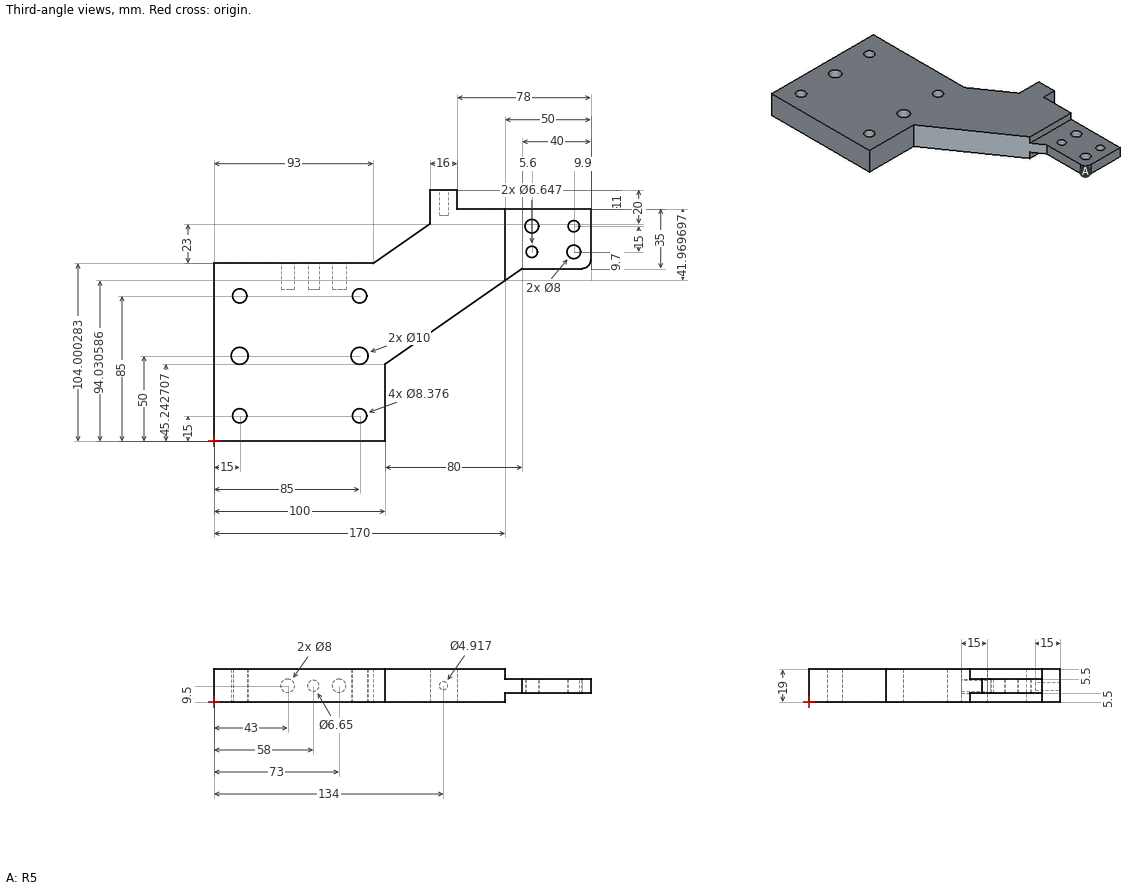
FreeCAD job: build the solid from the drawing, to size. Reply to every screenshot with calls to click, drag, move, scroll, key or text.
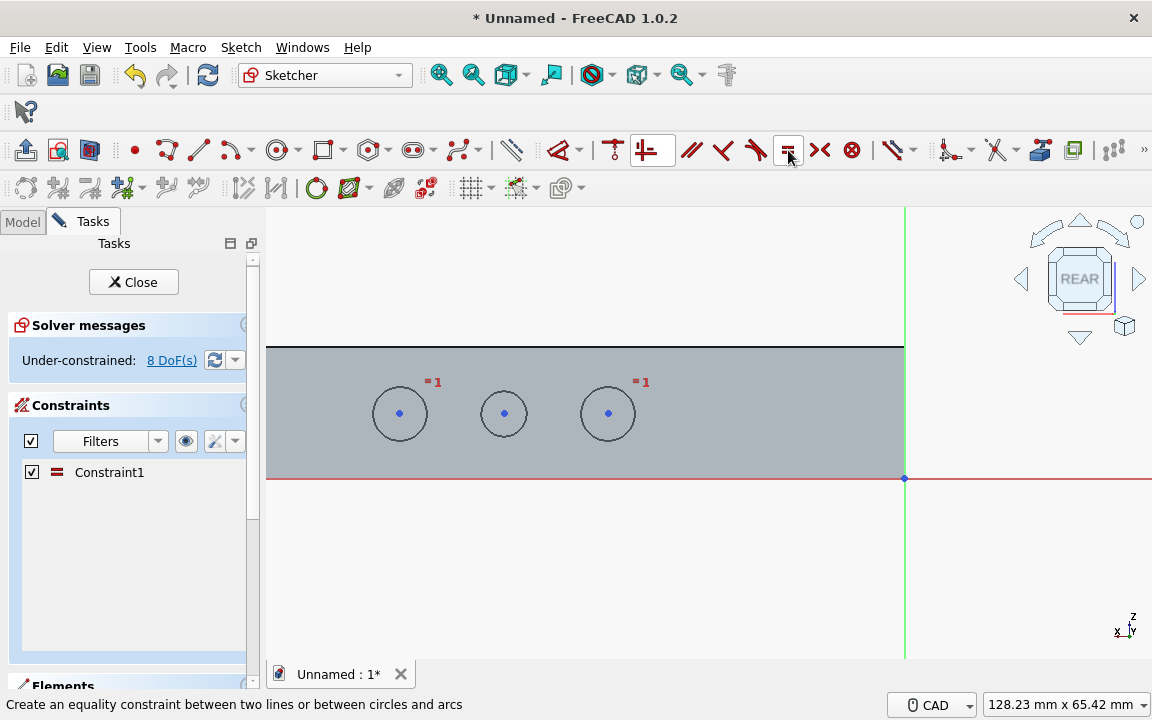
click(558, 150)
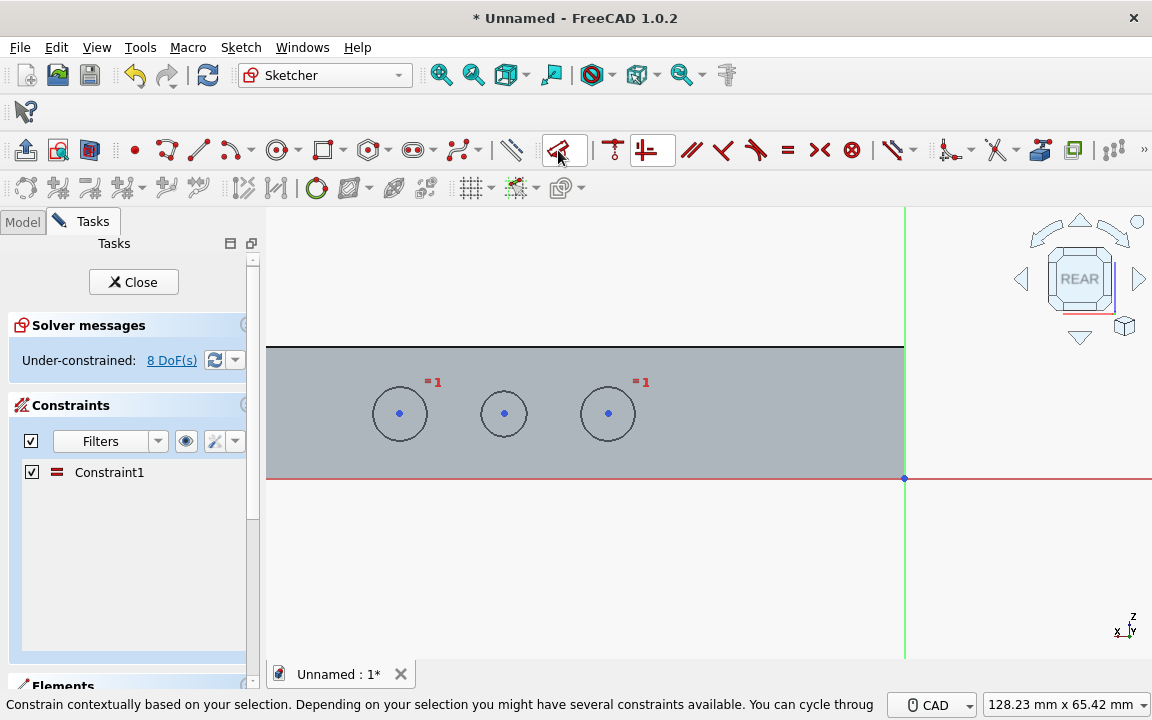
click(627, 395)
click(650, 372)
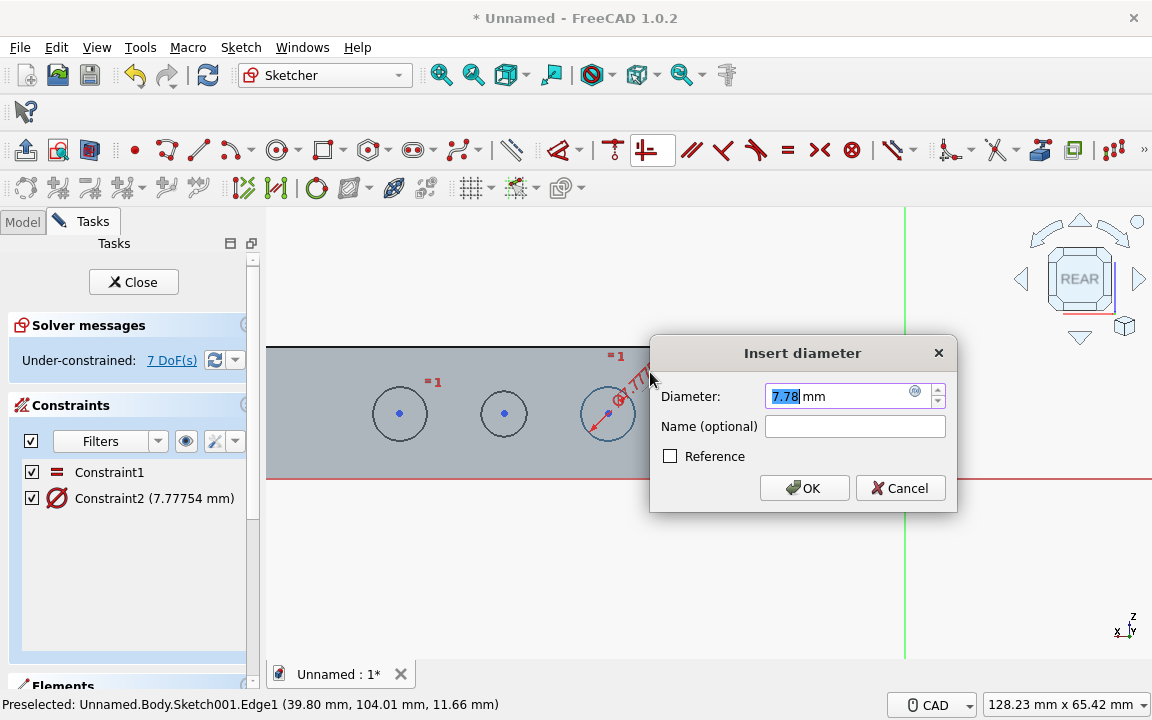
text(8)
key(Return)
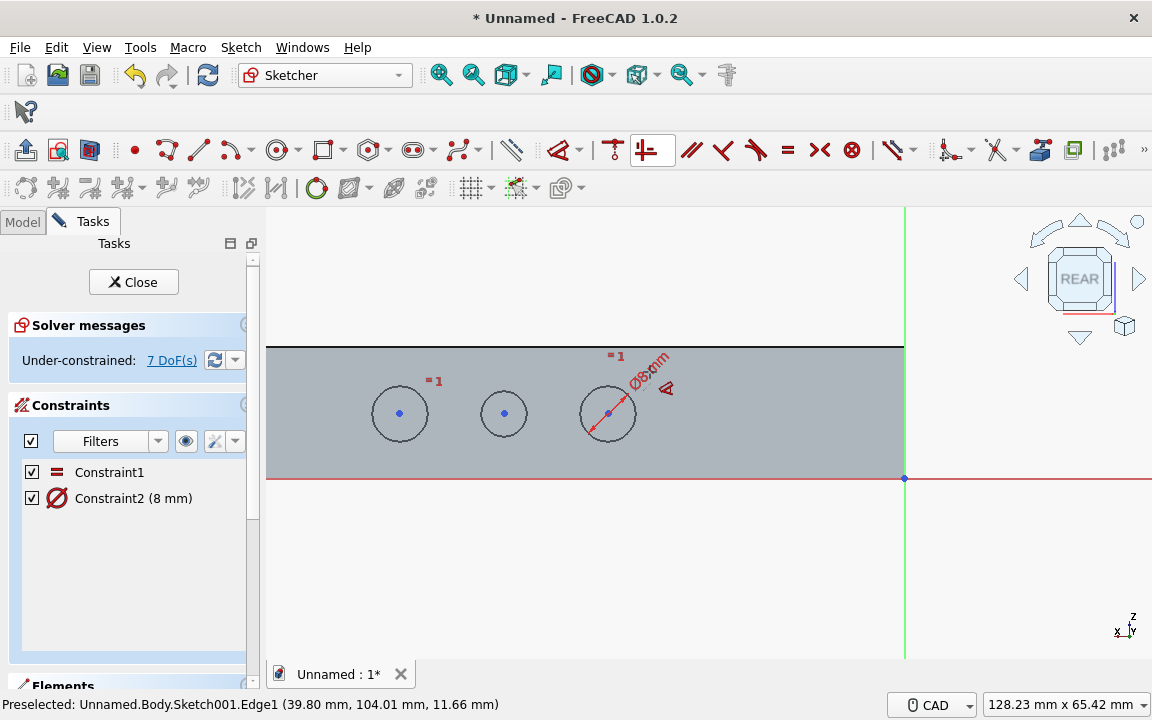
click(520, 398)
click(543, 375)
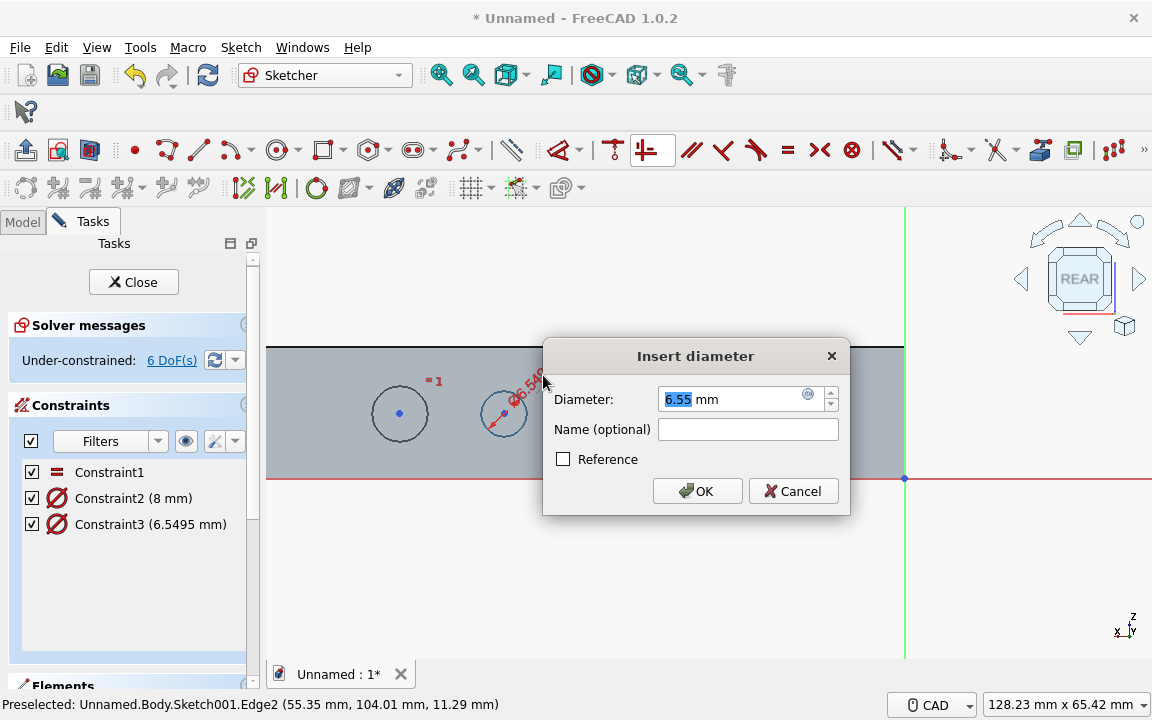
text(6.65)
key(Return)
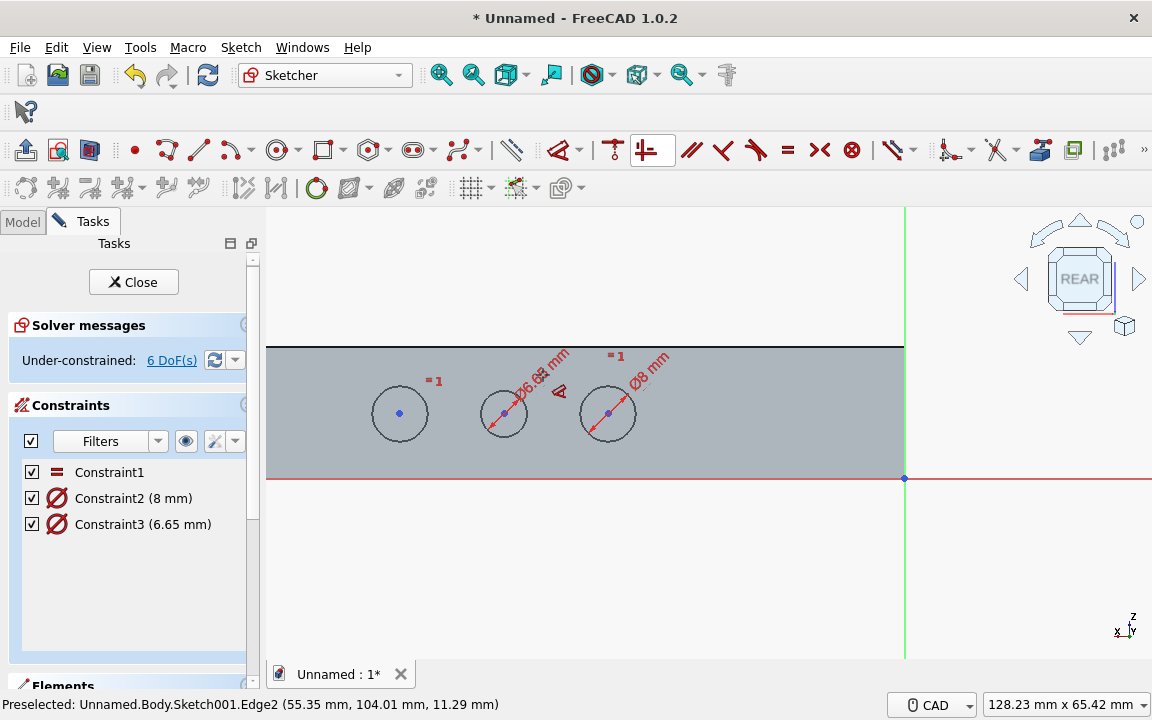
click(608, 414)
click(756, 513)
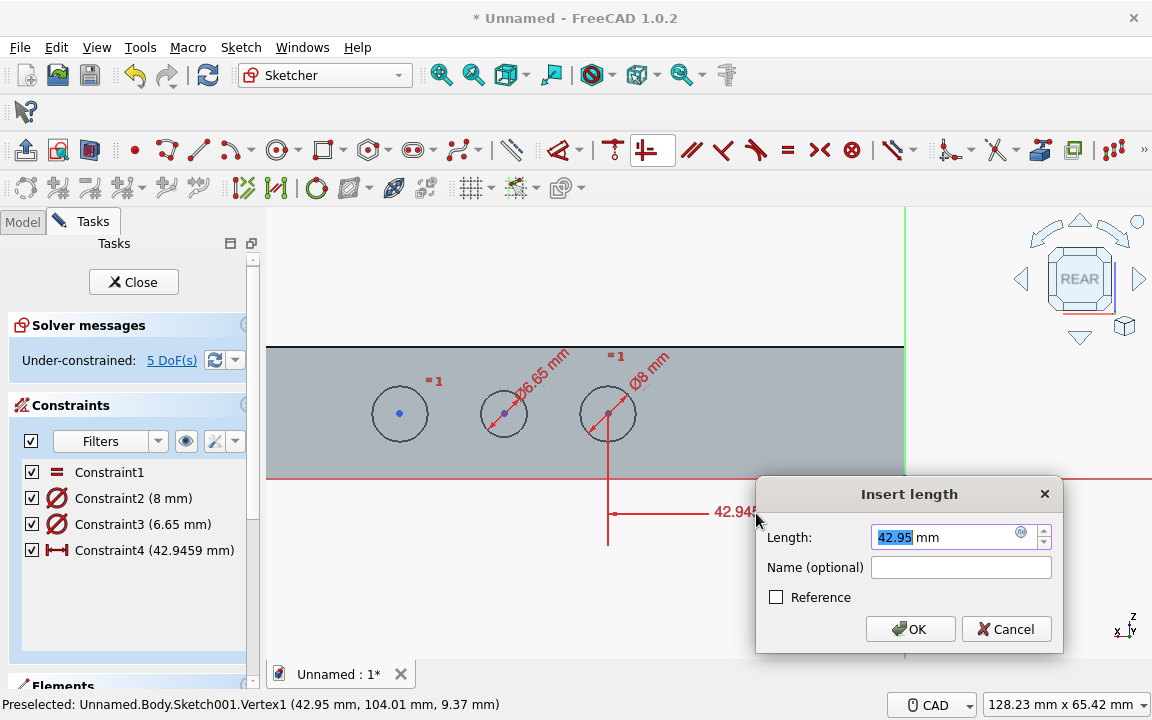
text(43)
key(Return)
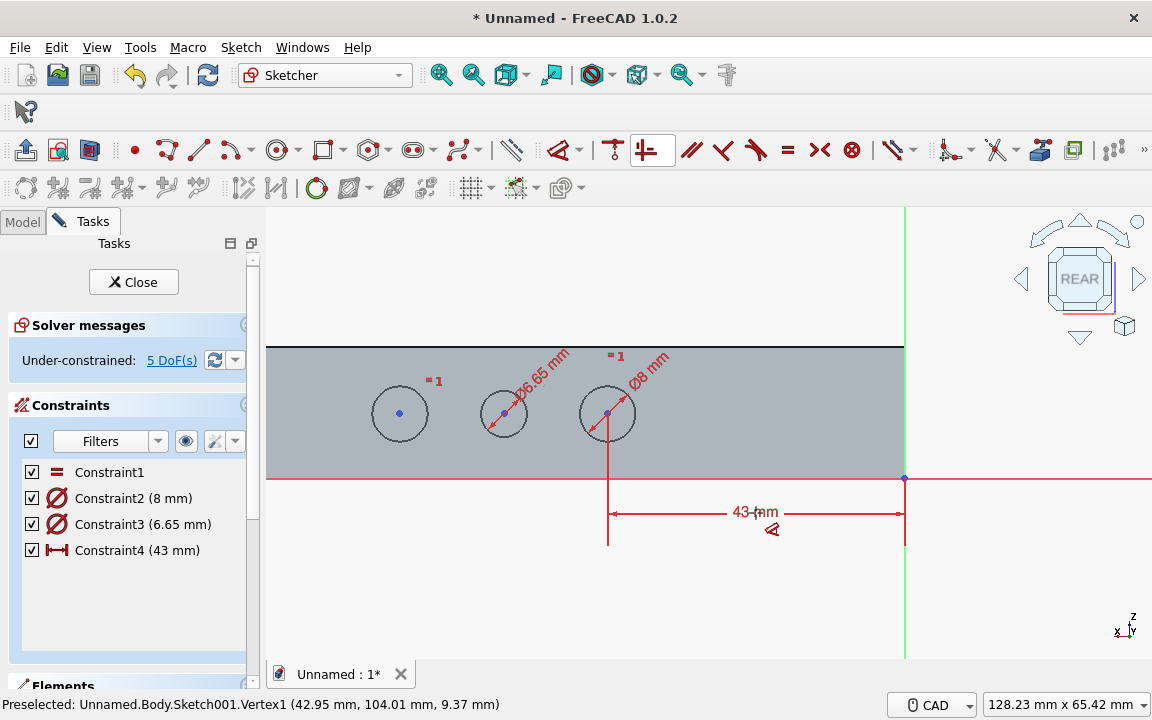
click(504, 414)
click(612, 513)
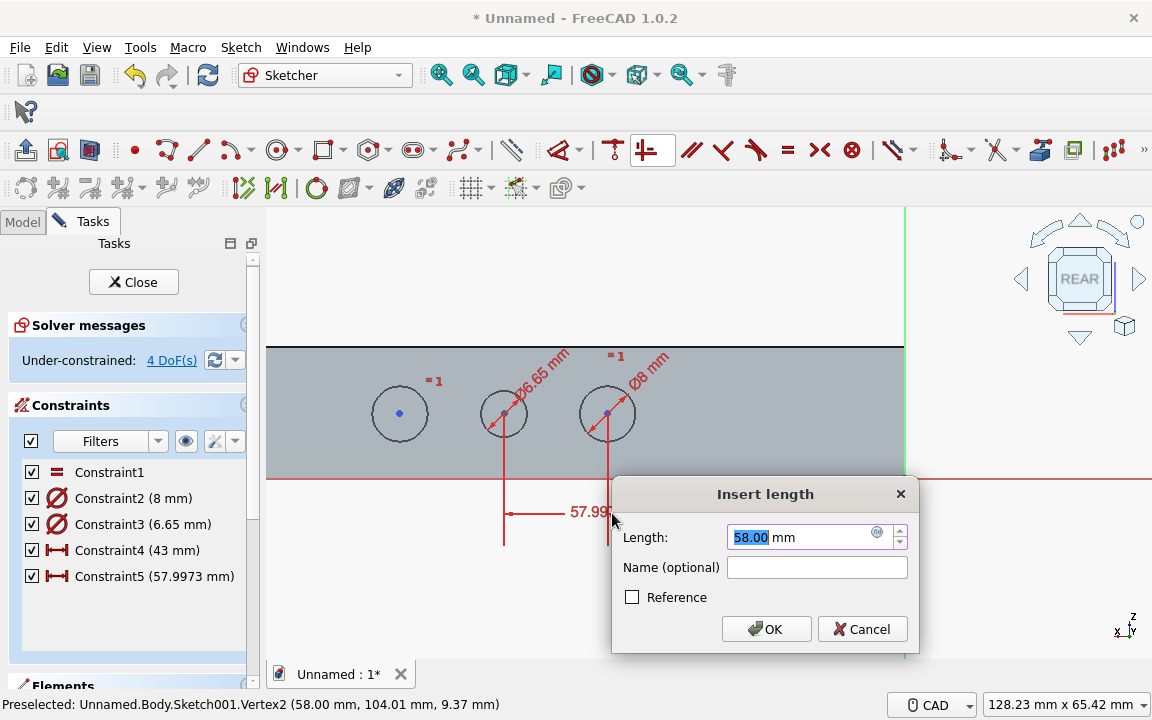
text(58)
key(Return)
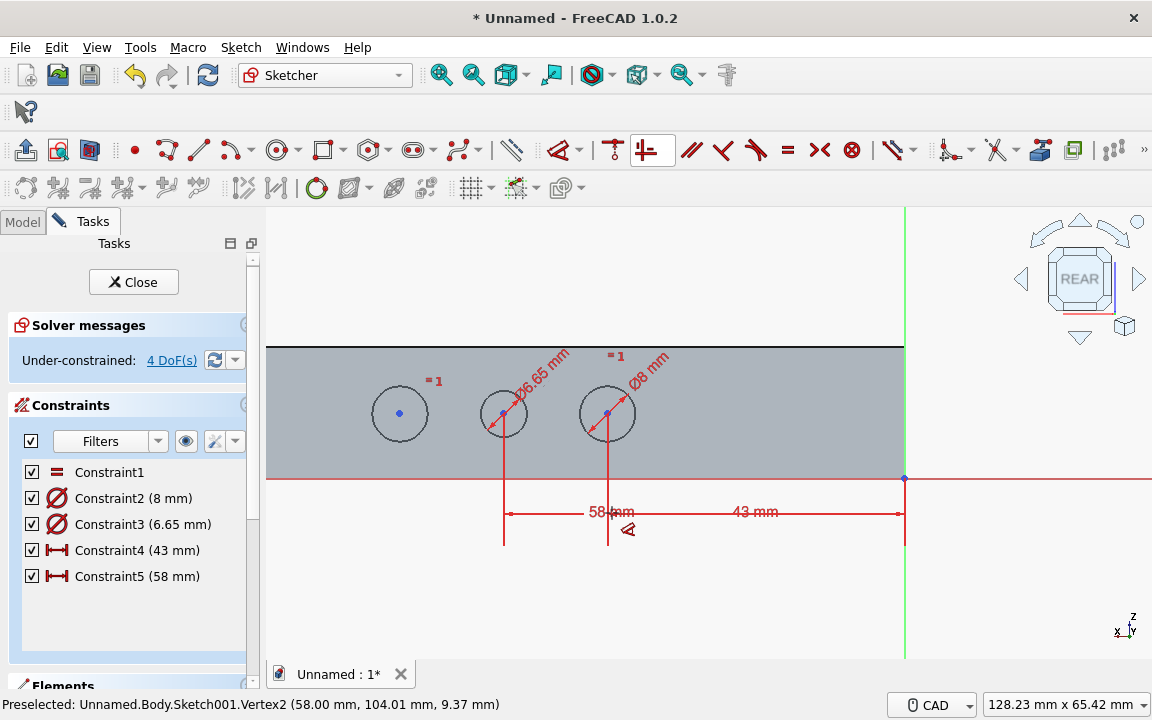
click(400, 414)
click(536, 513)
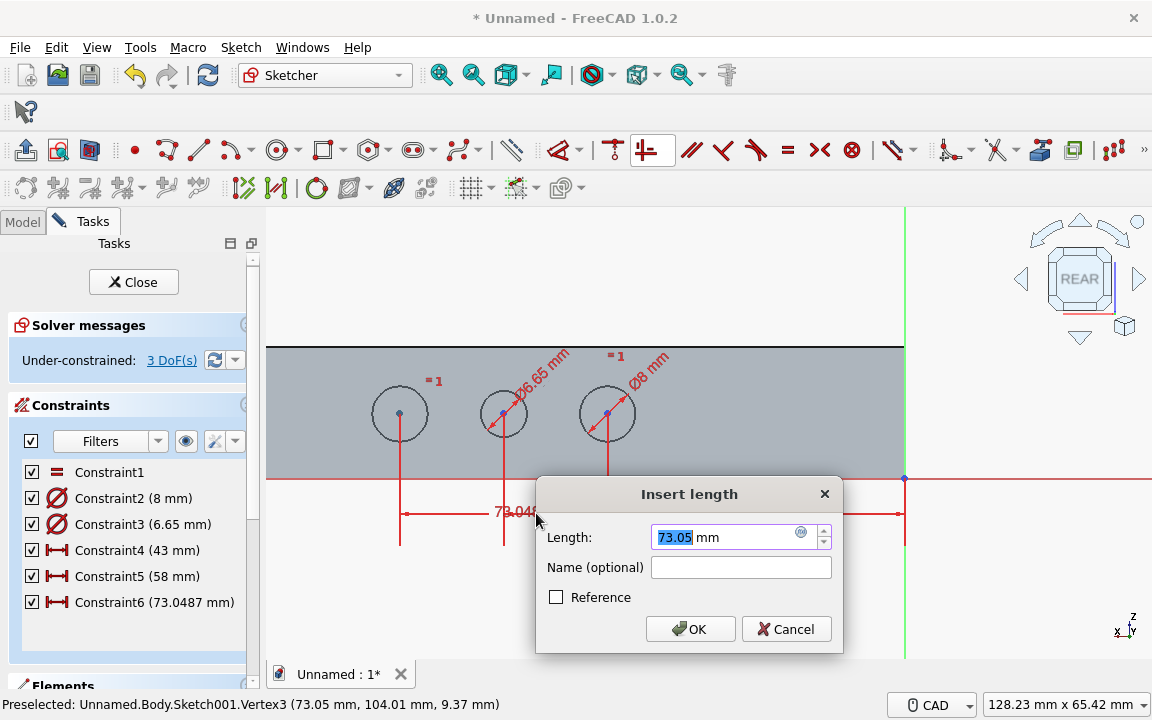
text(73)
key(Return)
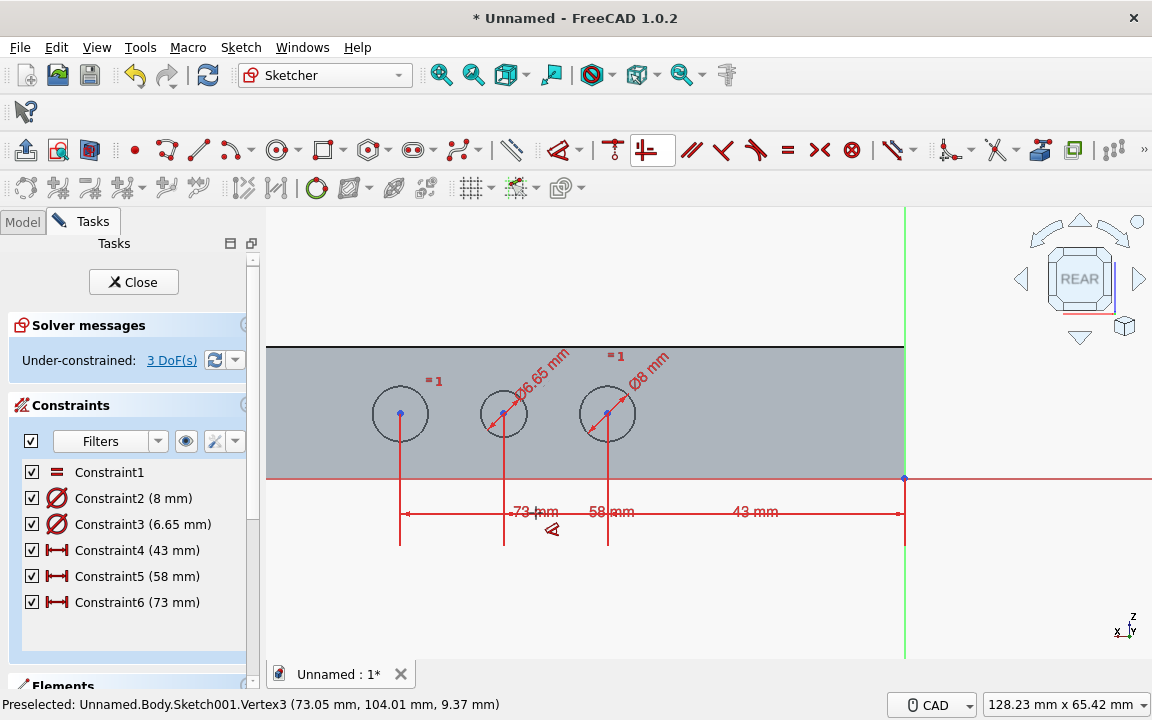
click(608, 414)
click(939, 446)